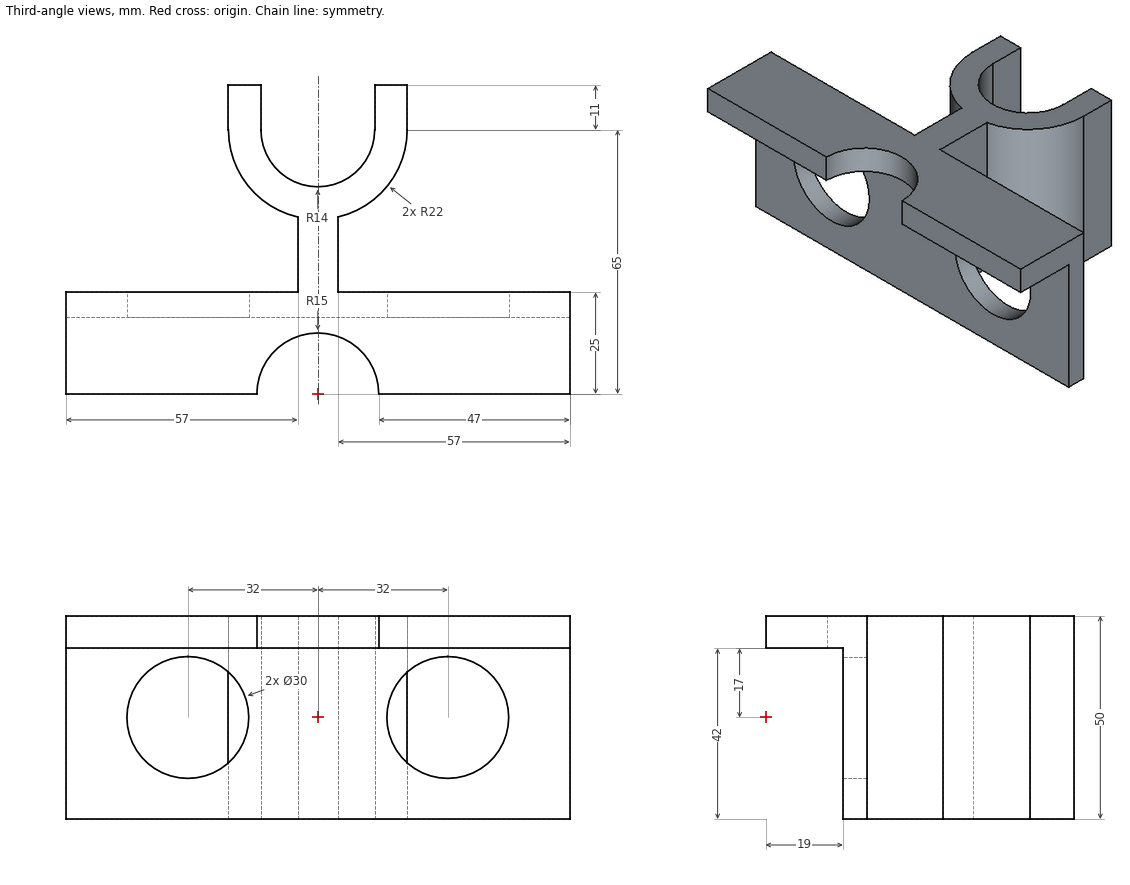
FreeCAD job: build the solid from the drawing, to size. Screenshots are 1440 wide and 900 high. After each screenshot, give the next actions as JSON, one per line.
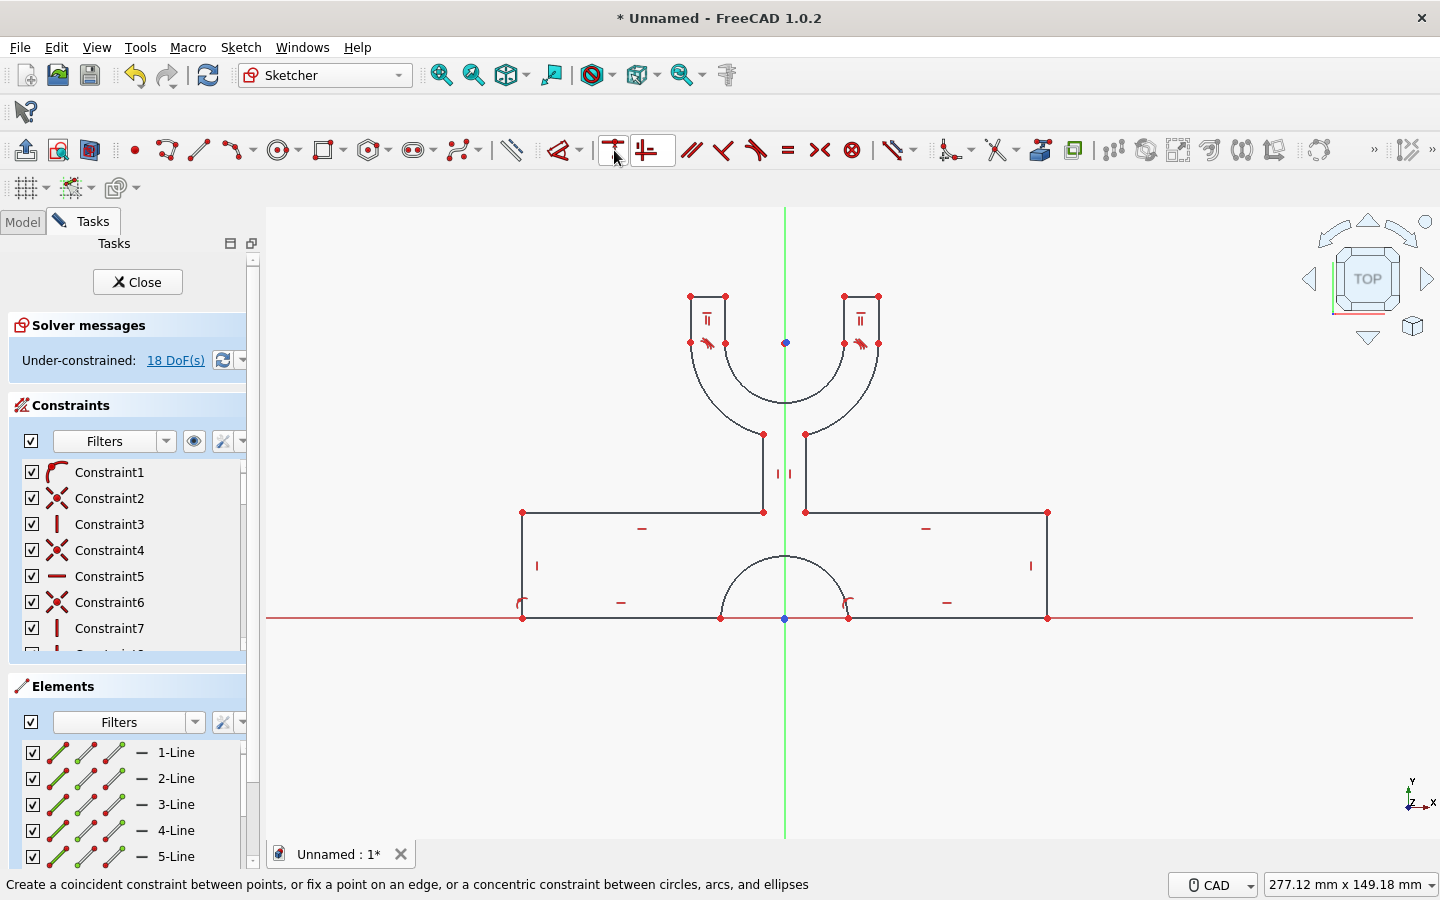
{"action": "left_click", "coordinate": [840, 419]}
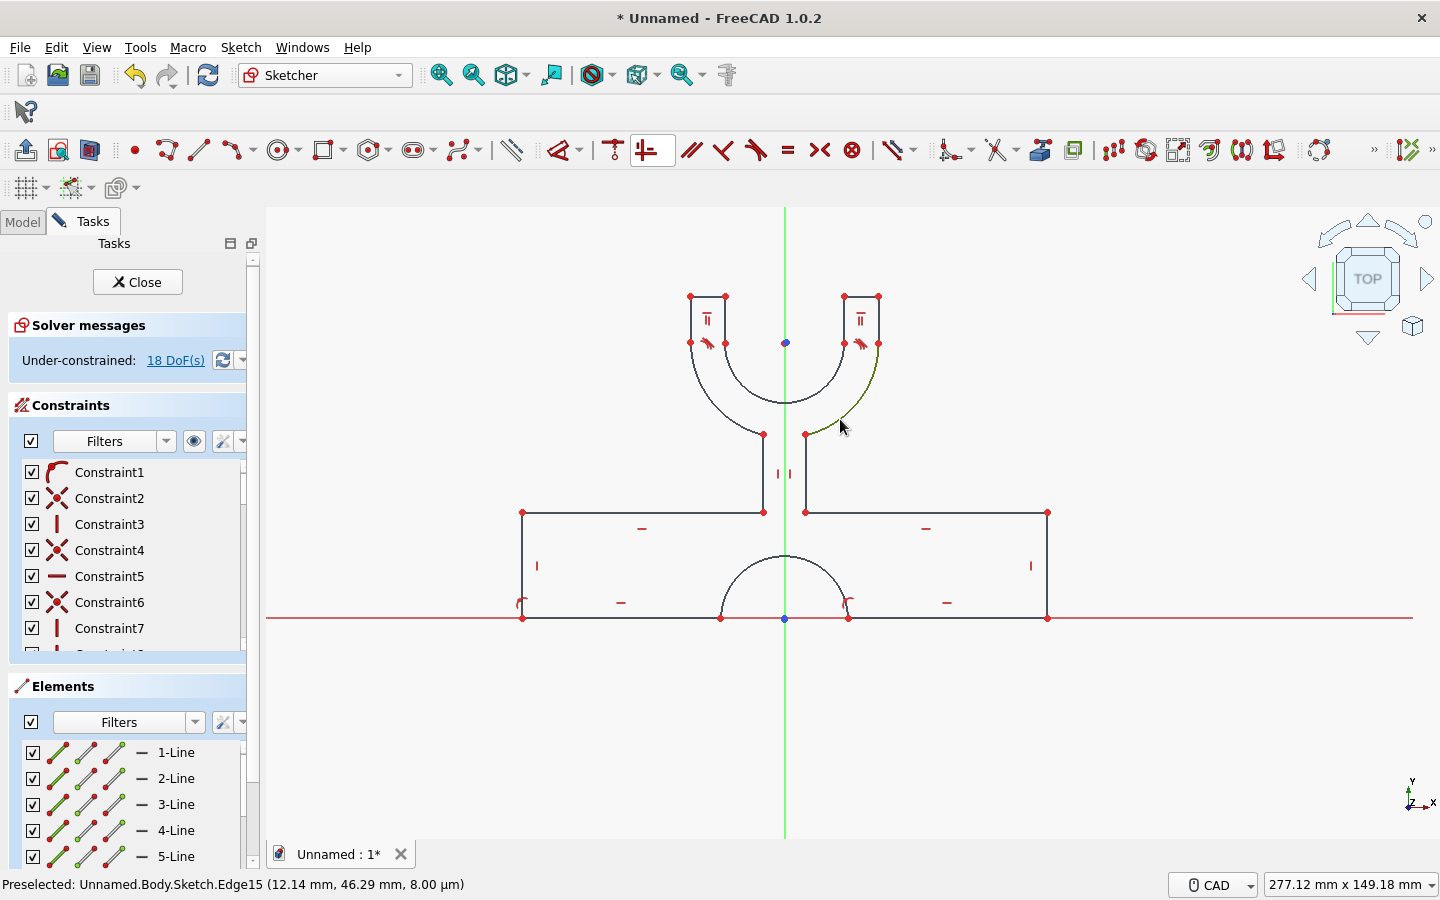
{"action": "left_click", "coordinate": [698, 379]}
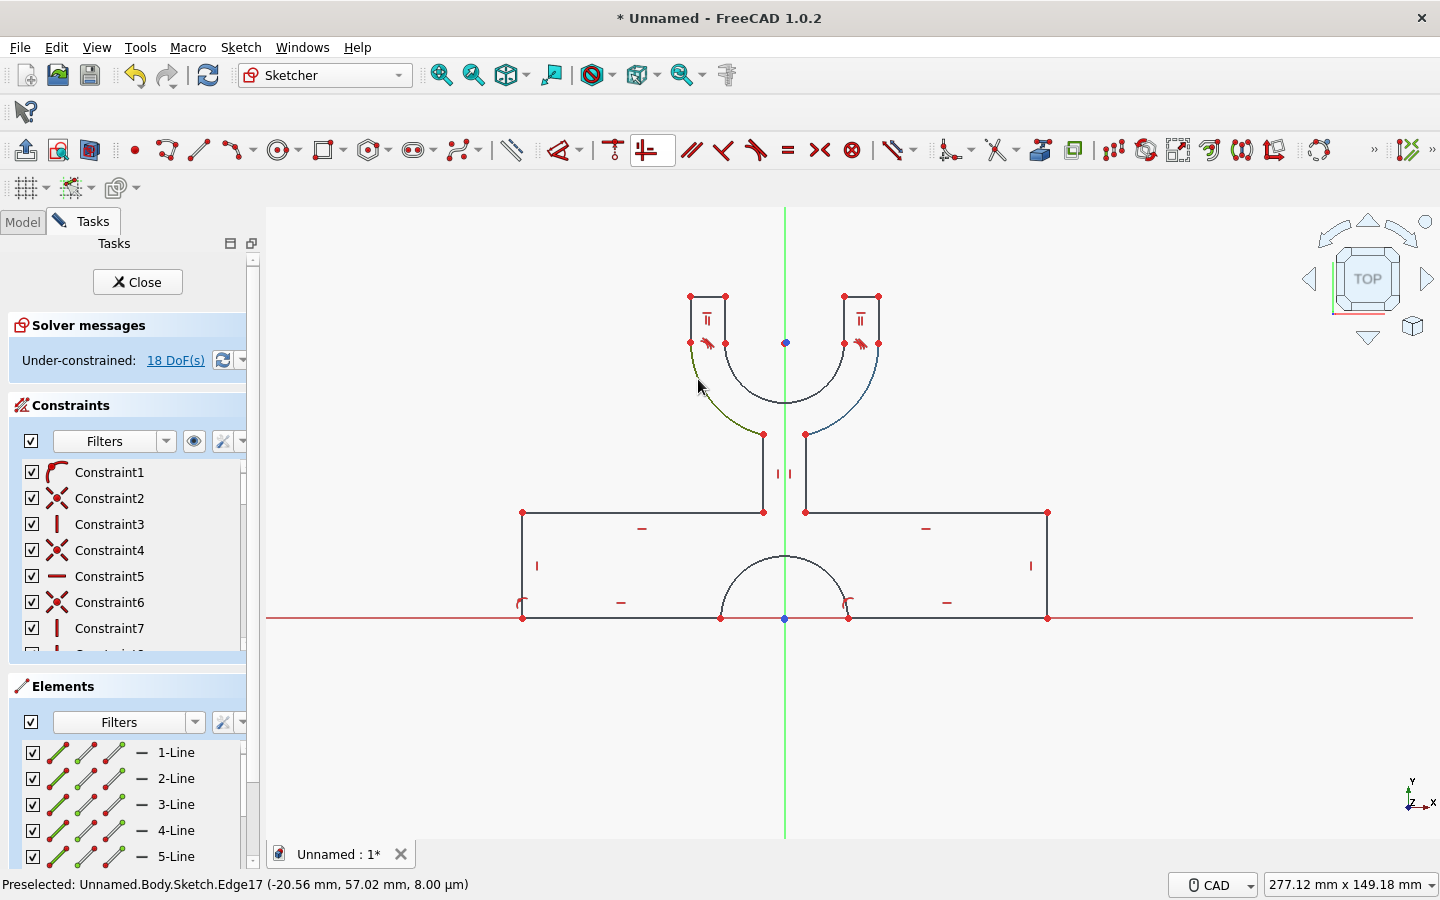
{"action": "left_click", "coordinate": [614, 150]}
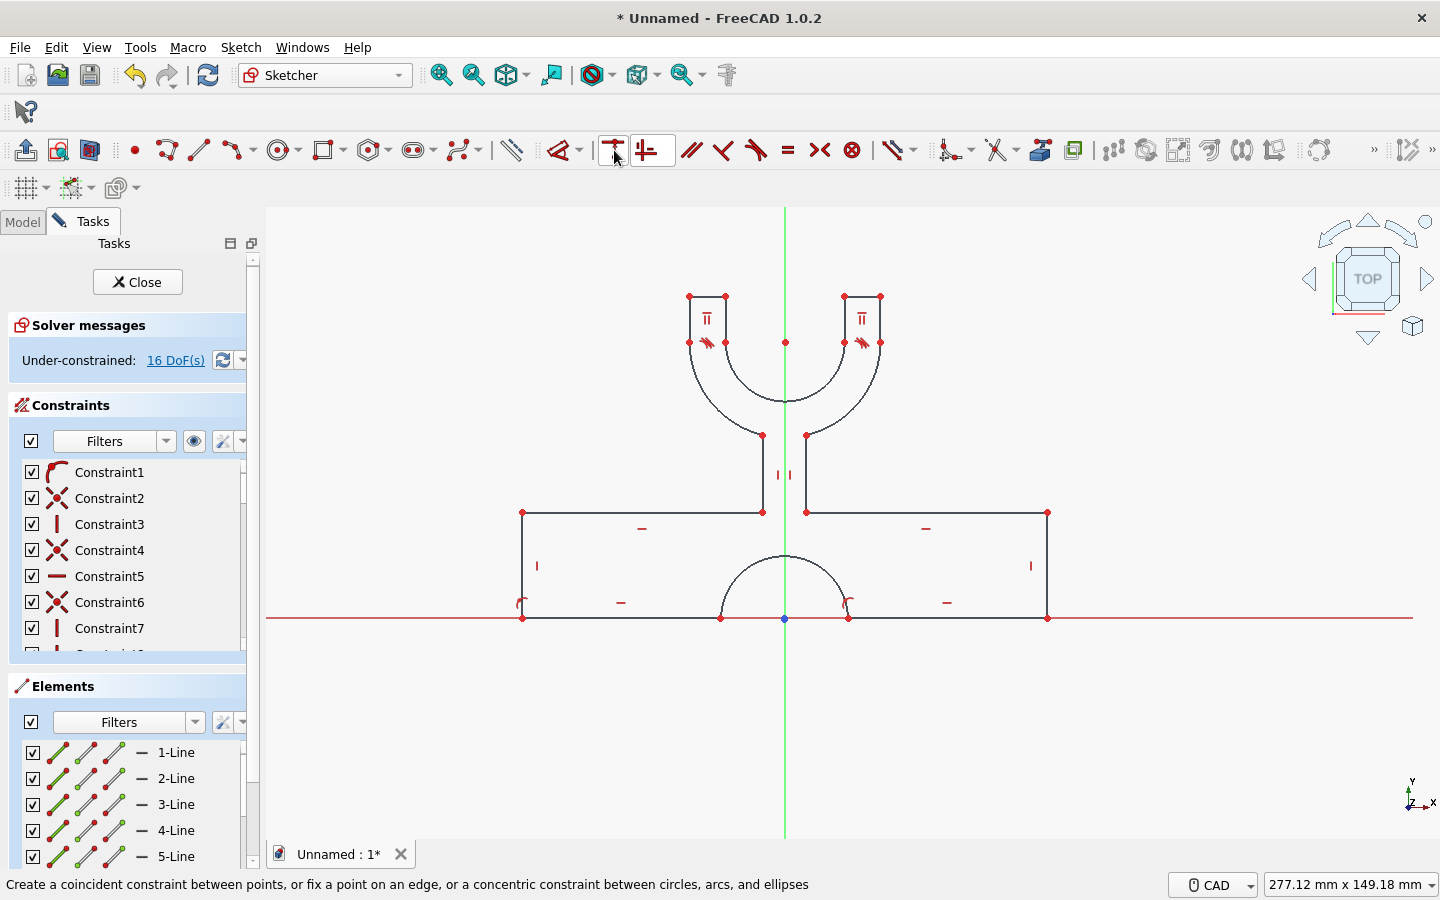
{"action": "left_click_drag", "start_coordinate": [774, 608], "coordinate": [795, 630]}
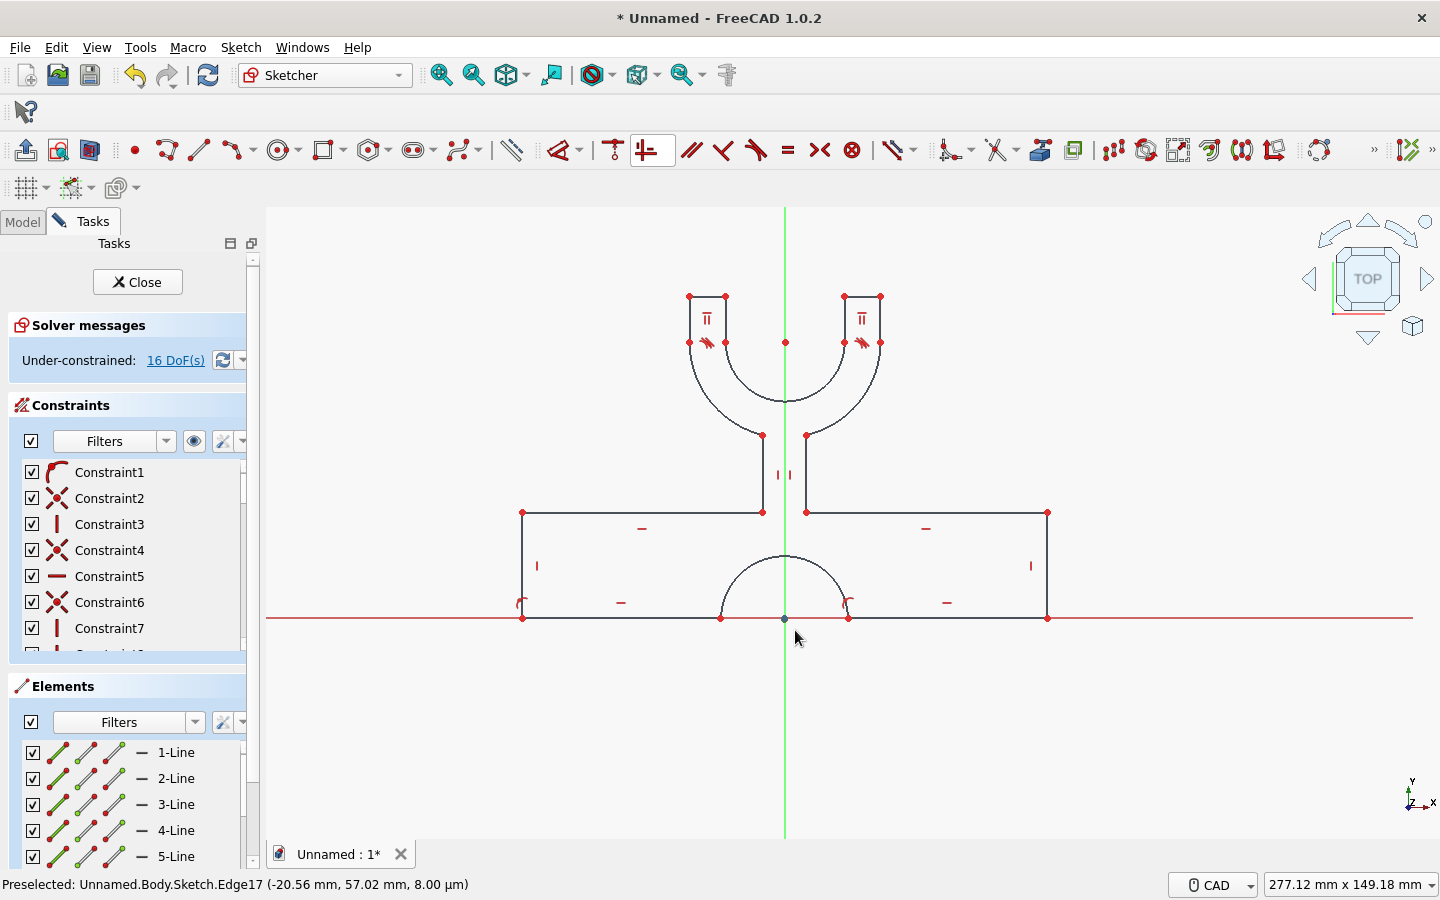
{"action": "left_click", "coordinate": [614, 150]}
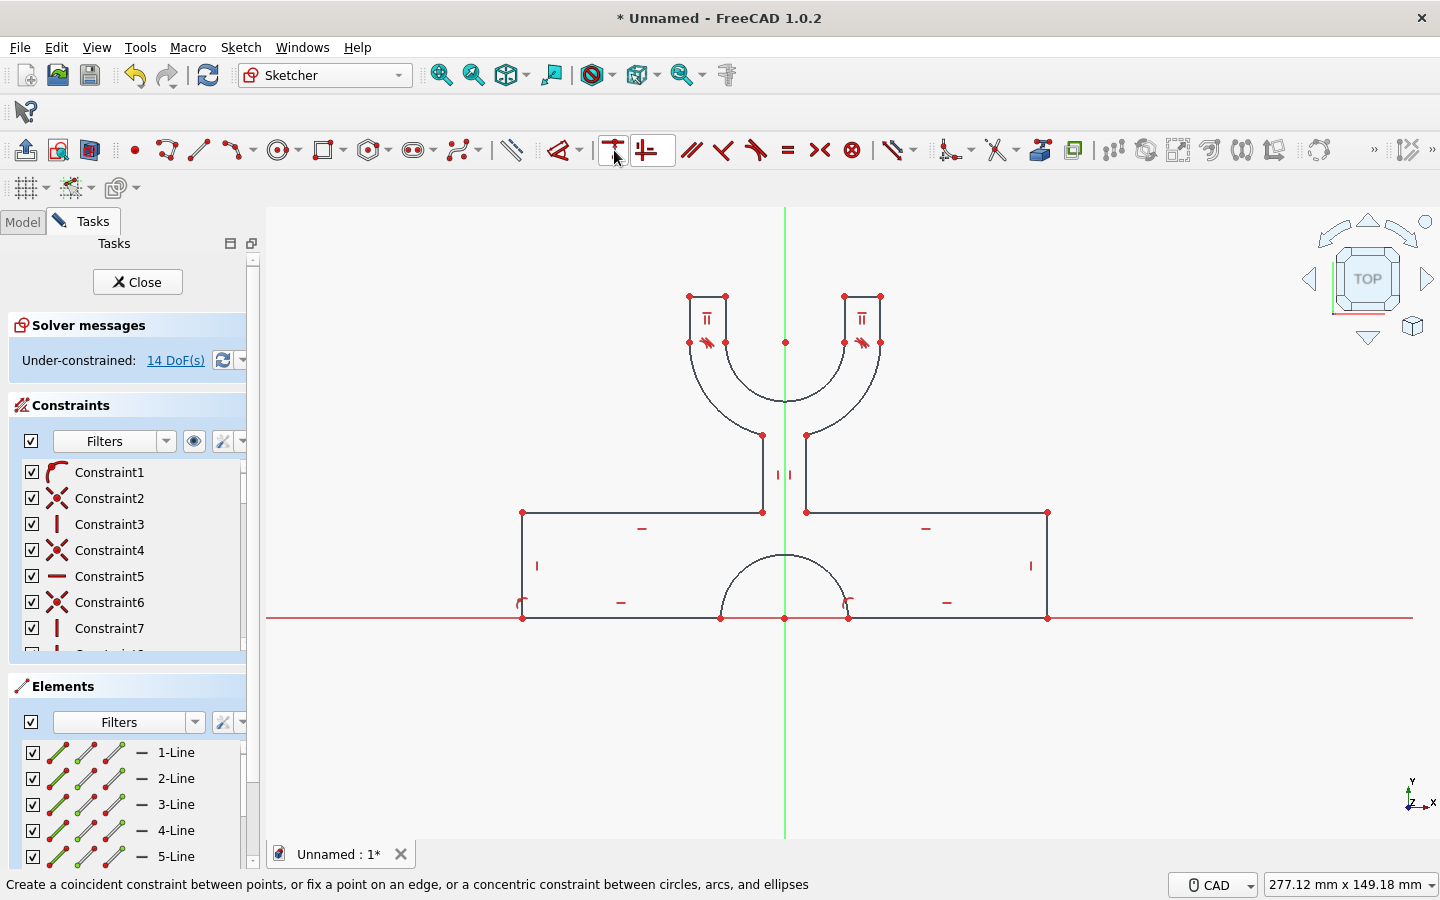
{"action": "left_click", "coordinate": [841, 419]}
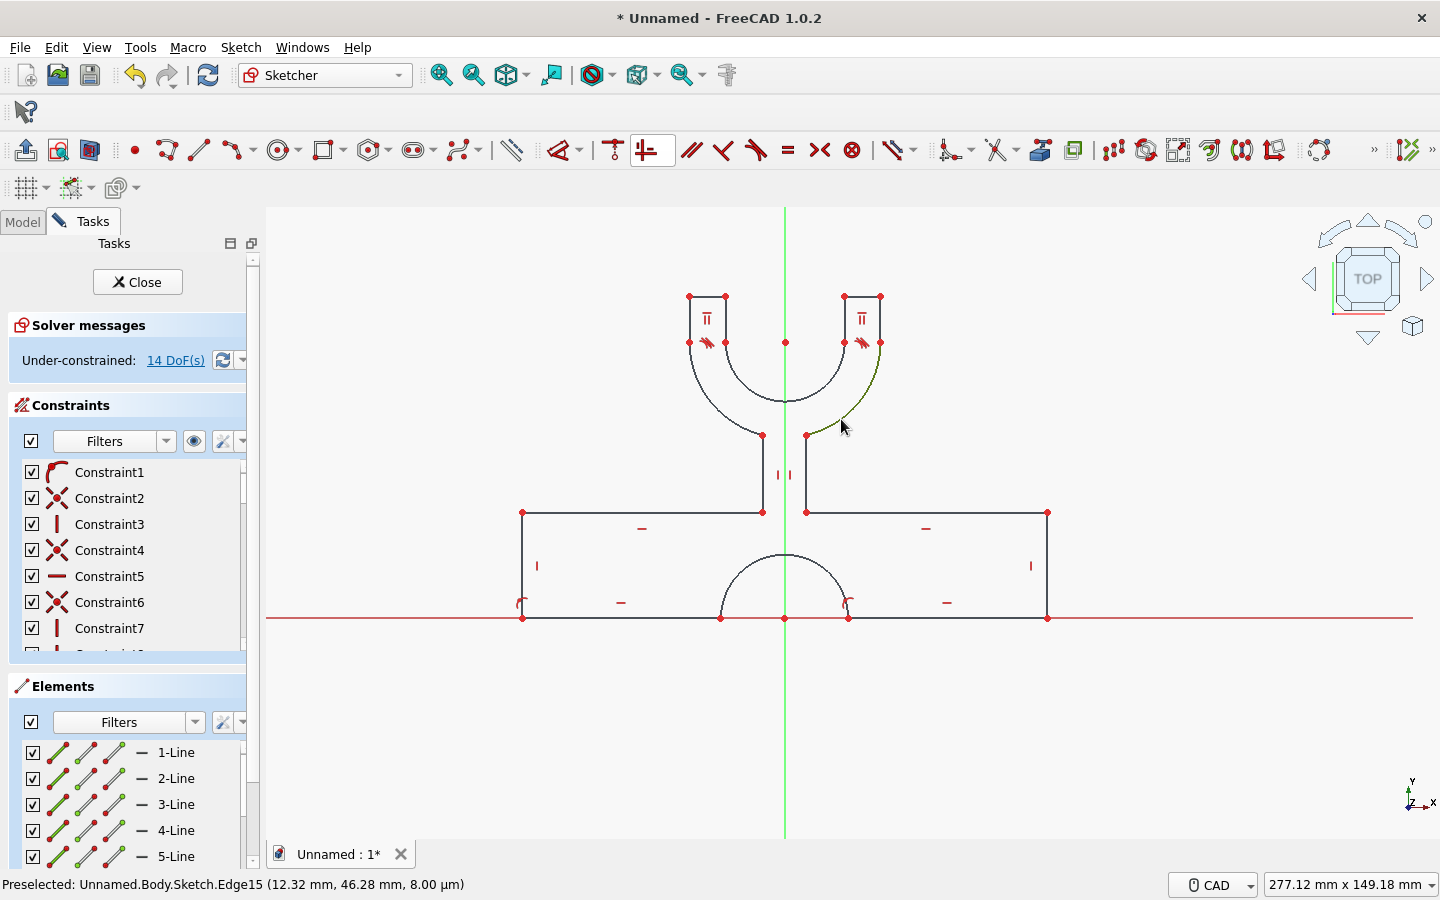
{"action": "left_click", "coordinate": [697, 379]}